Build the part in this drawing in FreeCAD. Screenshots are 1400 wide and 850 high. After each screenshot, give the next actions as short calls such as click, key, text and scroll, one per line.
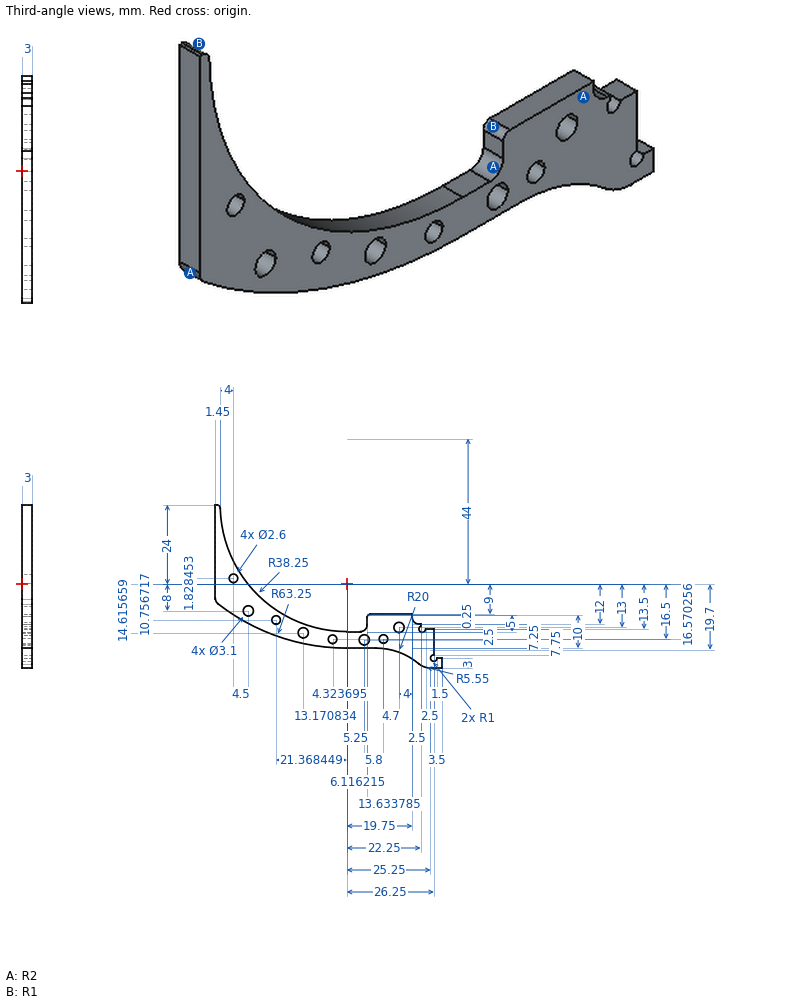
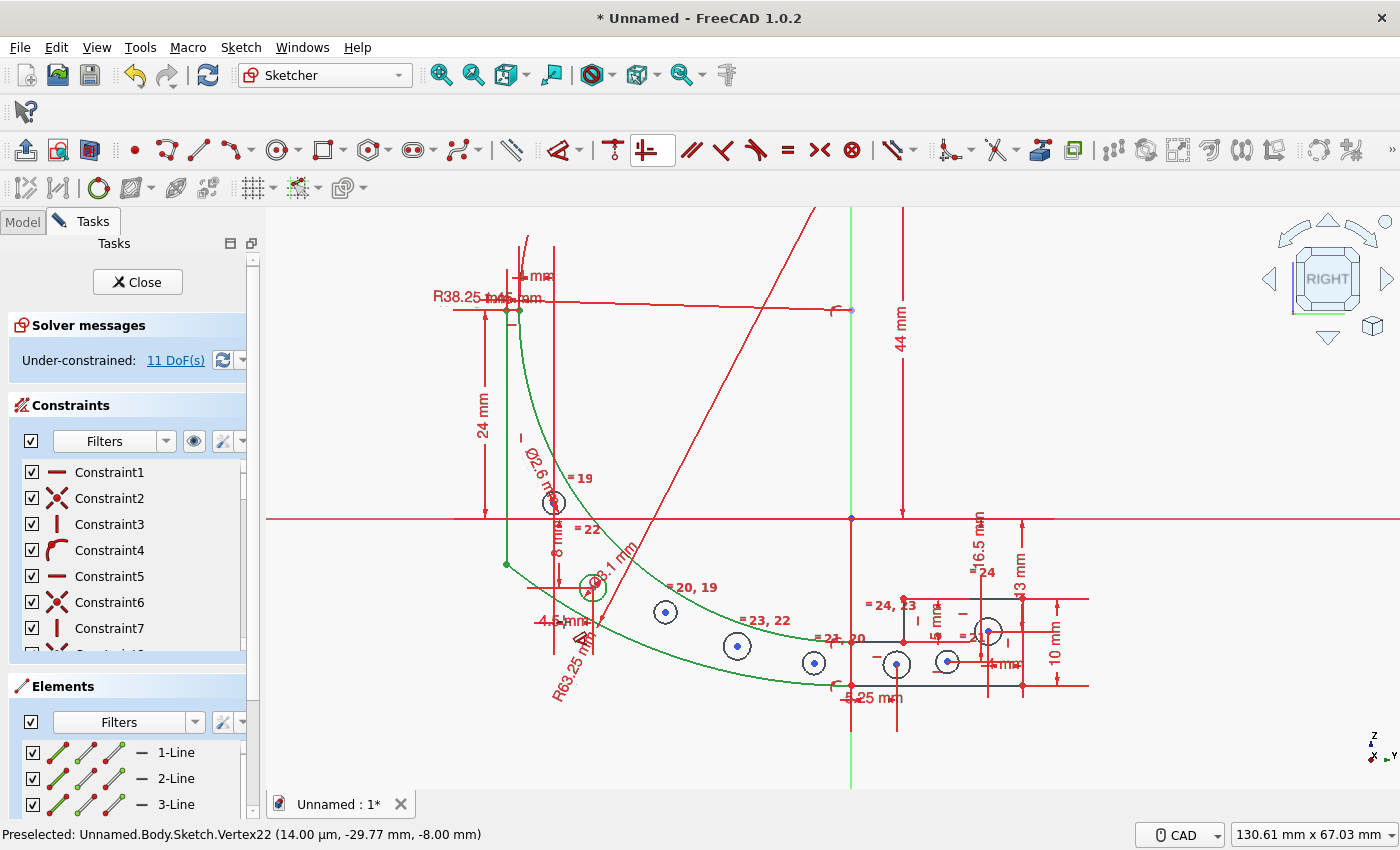
scroll(904, 642, up, 4)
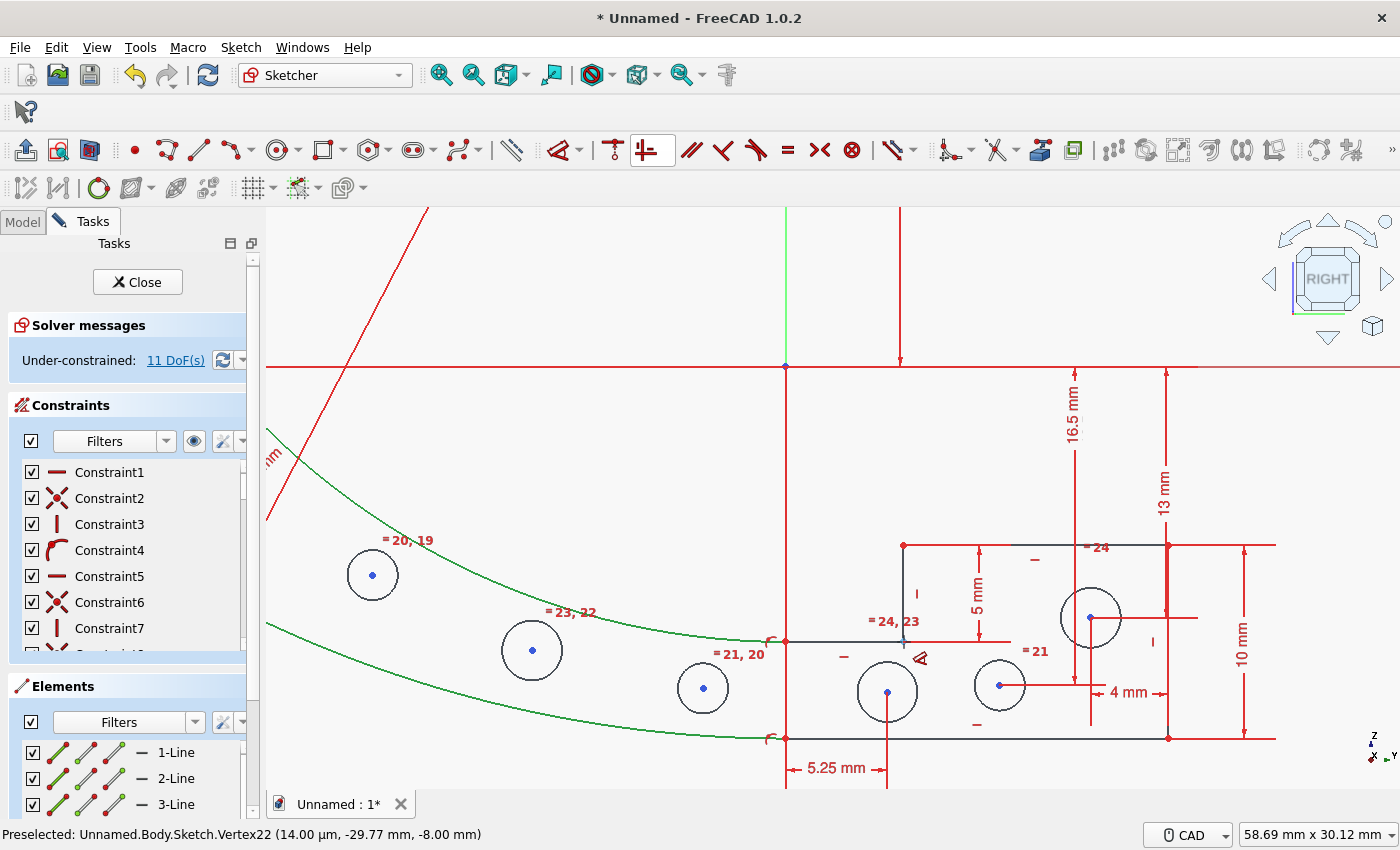
click(903, 642)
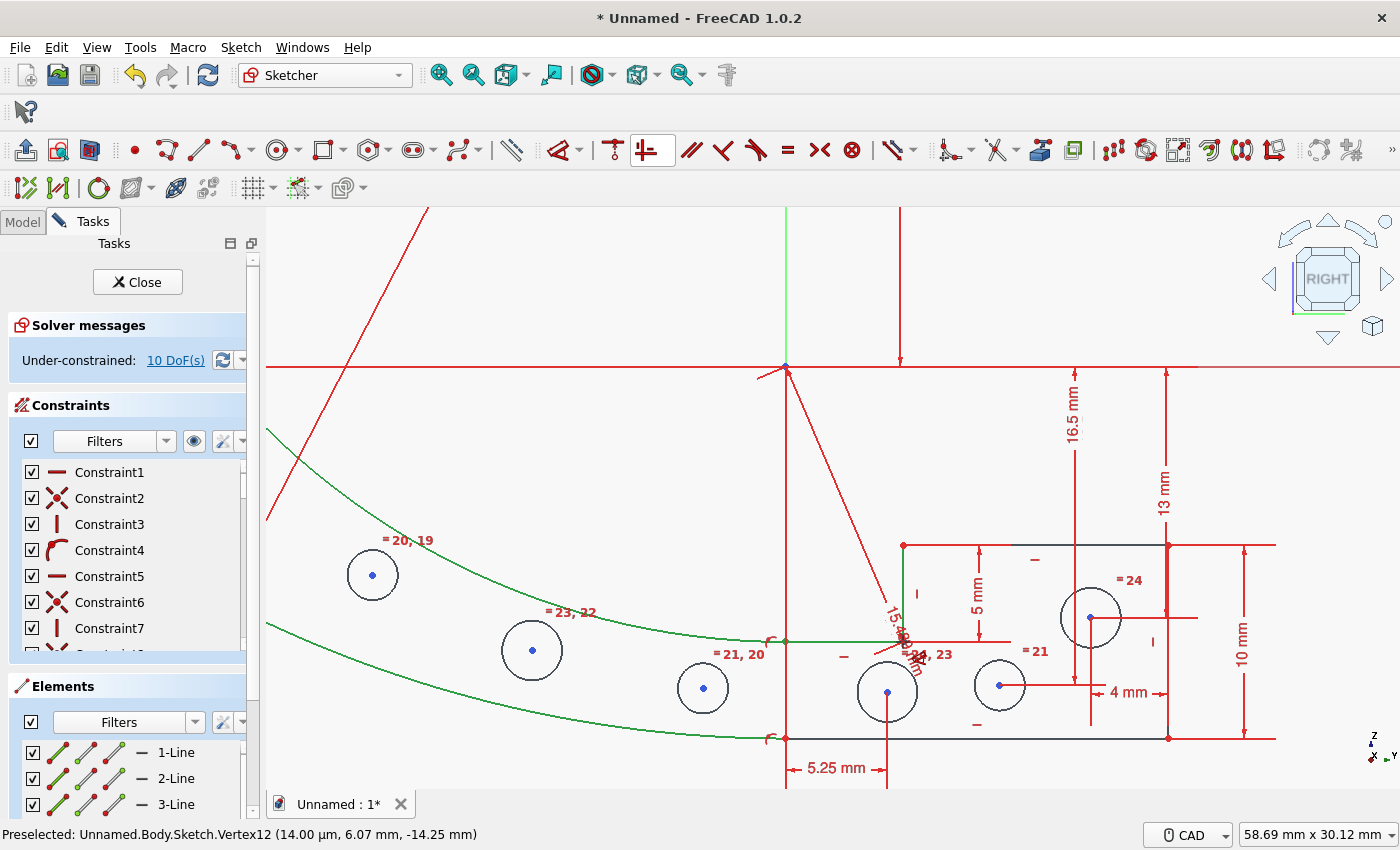
click(887, 692)
click(937, 667)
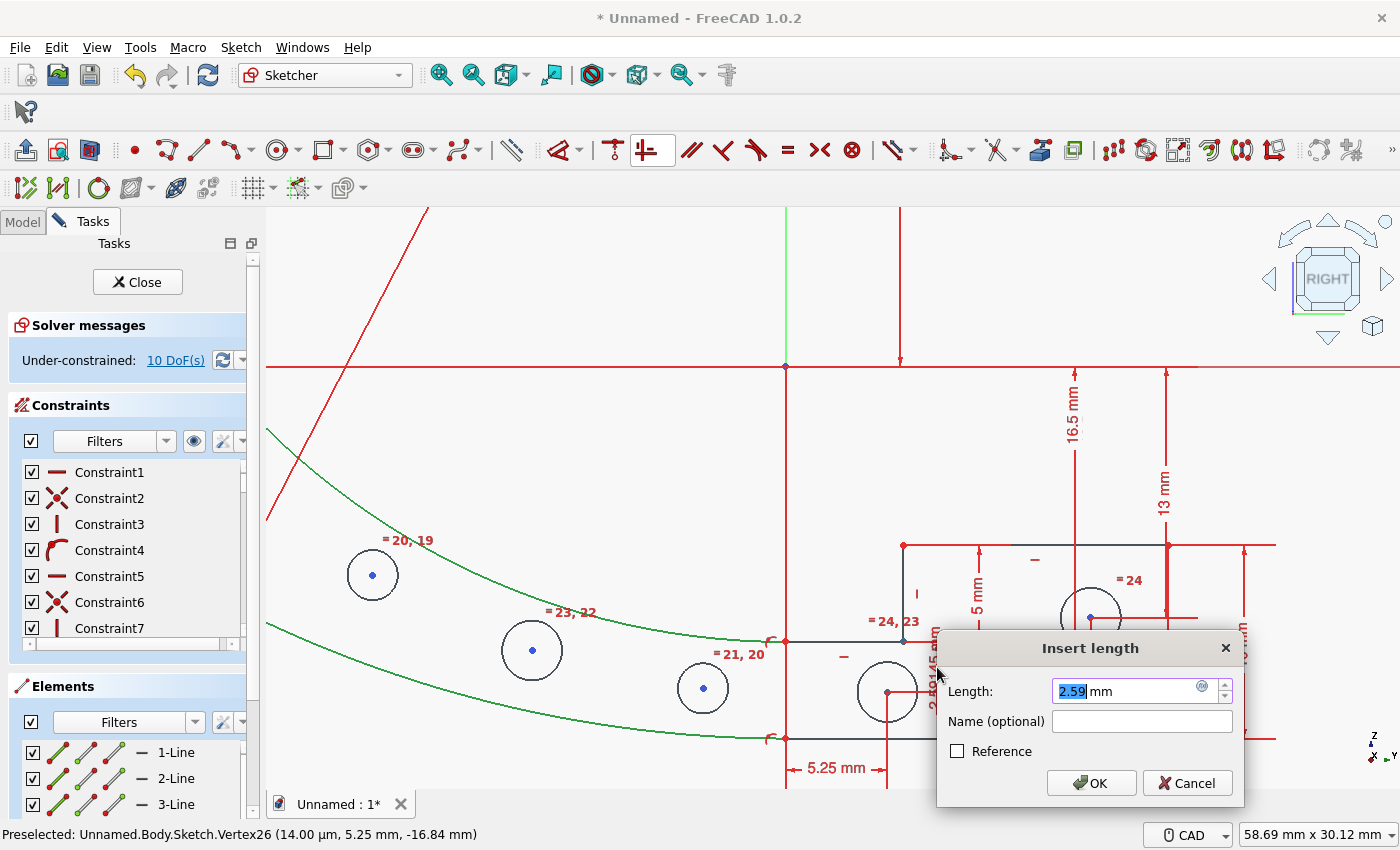
text(2.5)
key(Return)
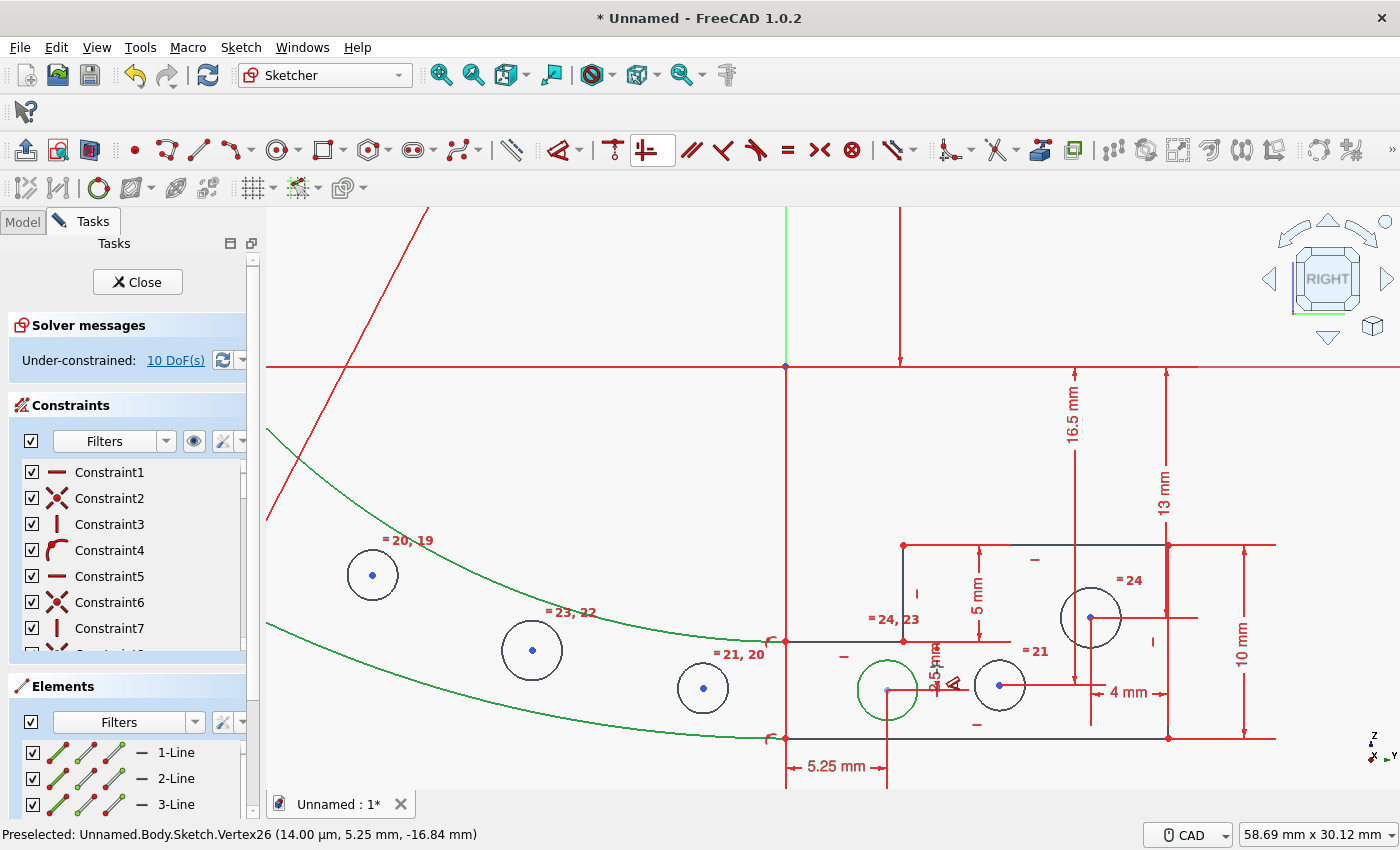
click(887, 690)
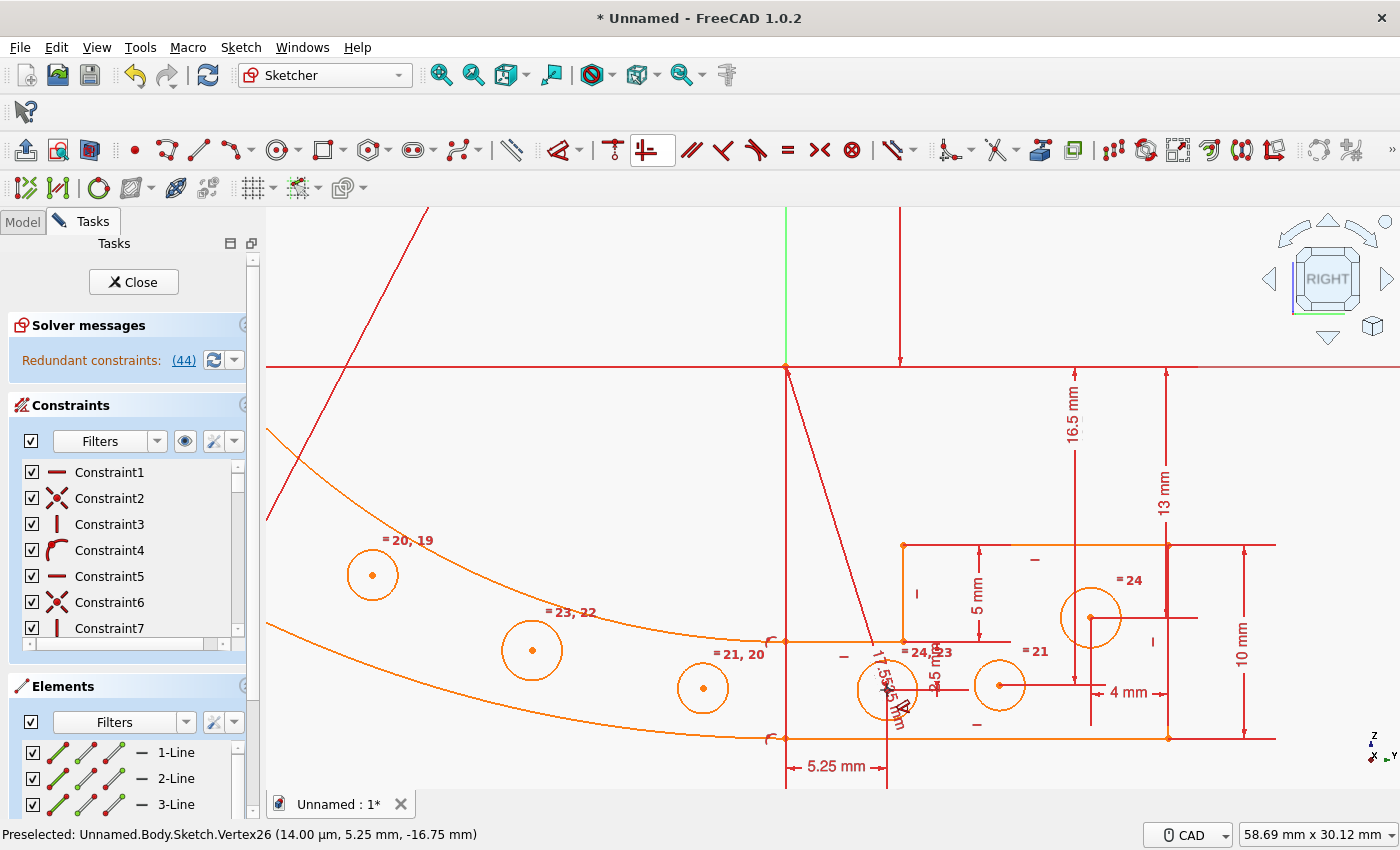
click(1000, 685)
click(944, 724)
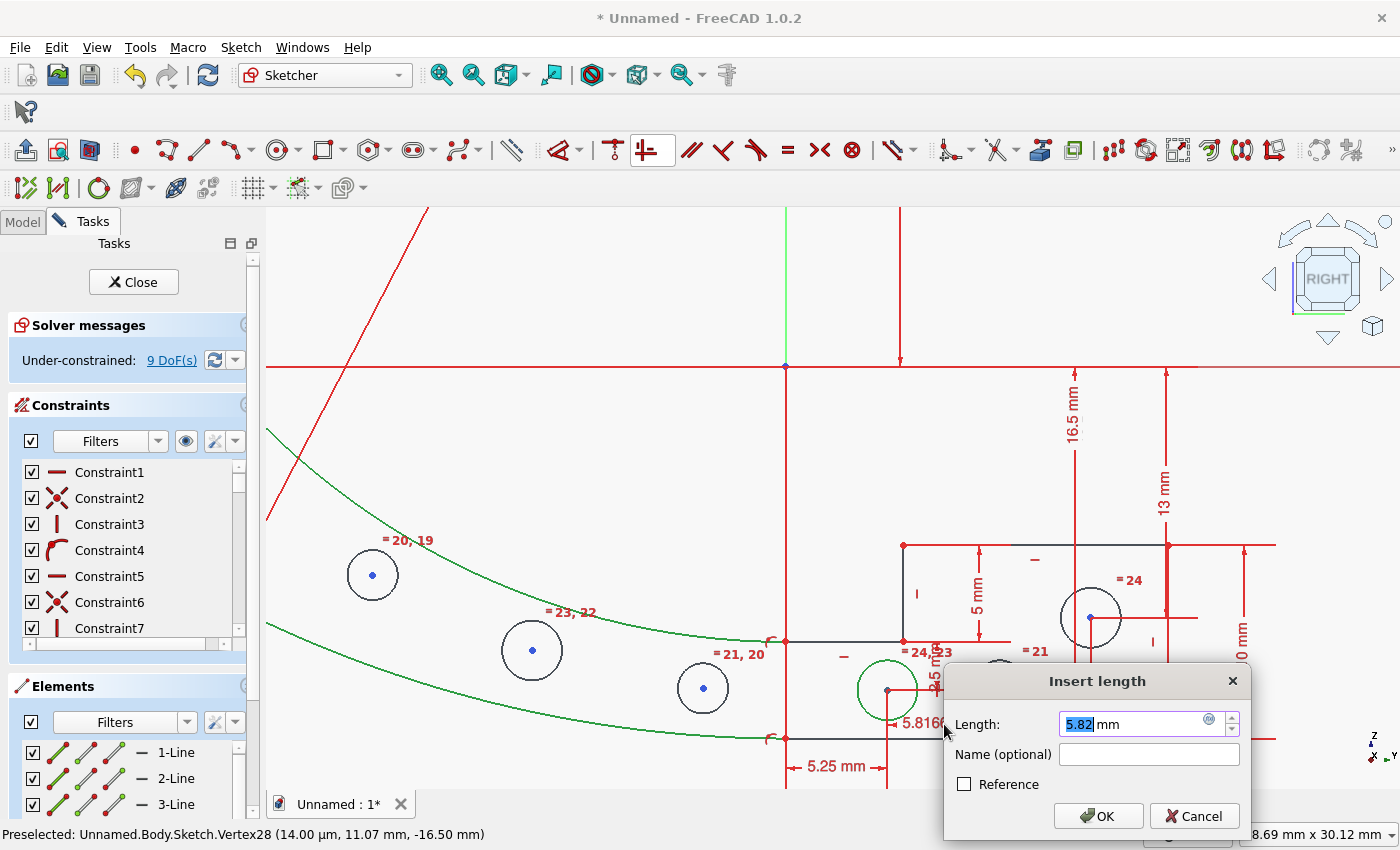
text(5.8)
key(Return)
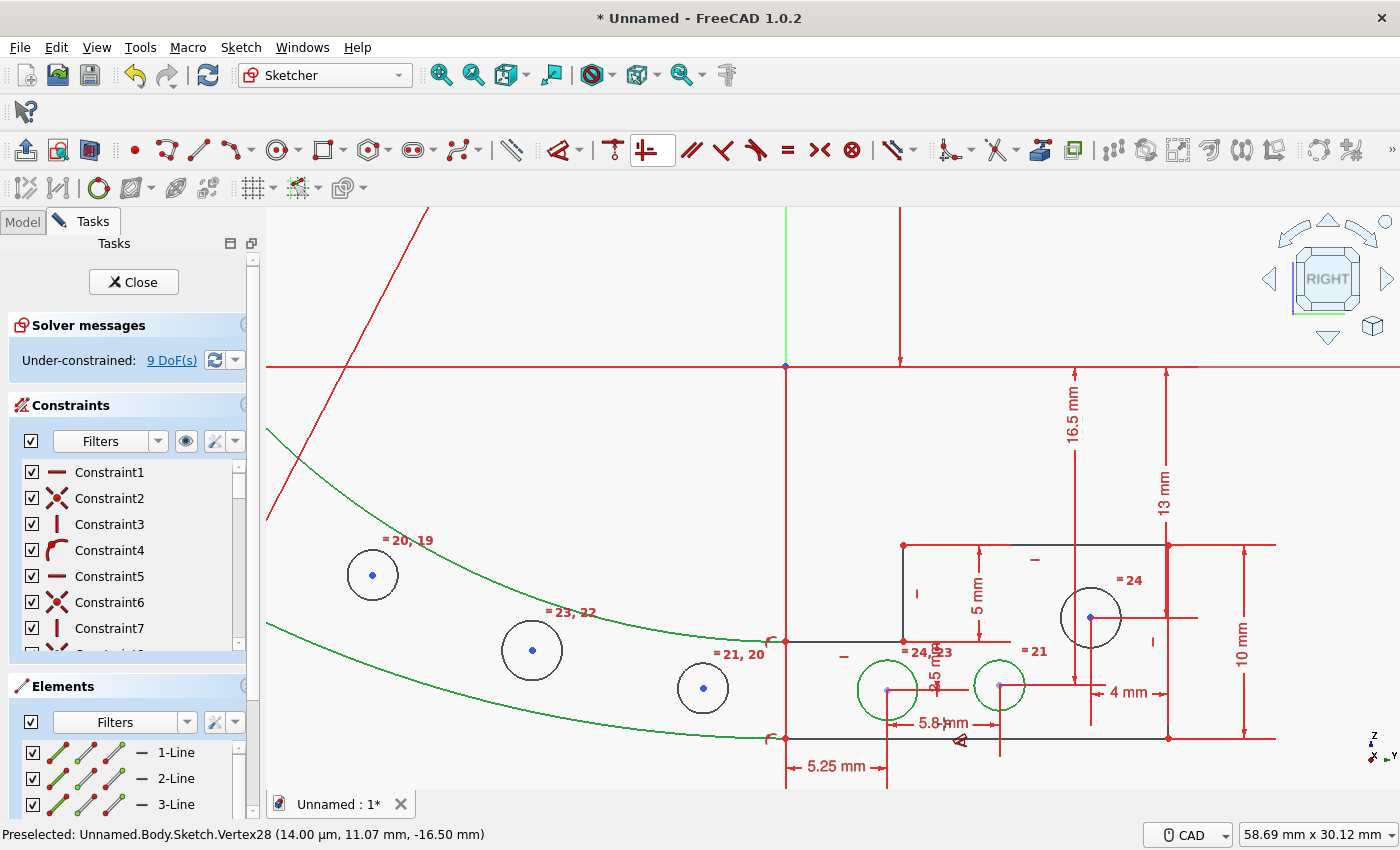
click(1091, 618)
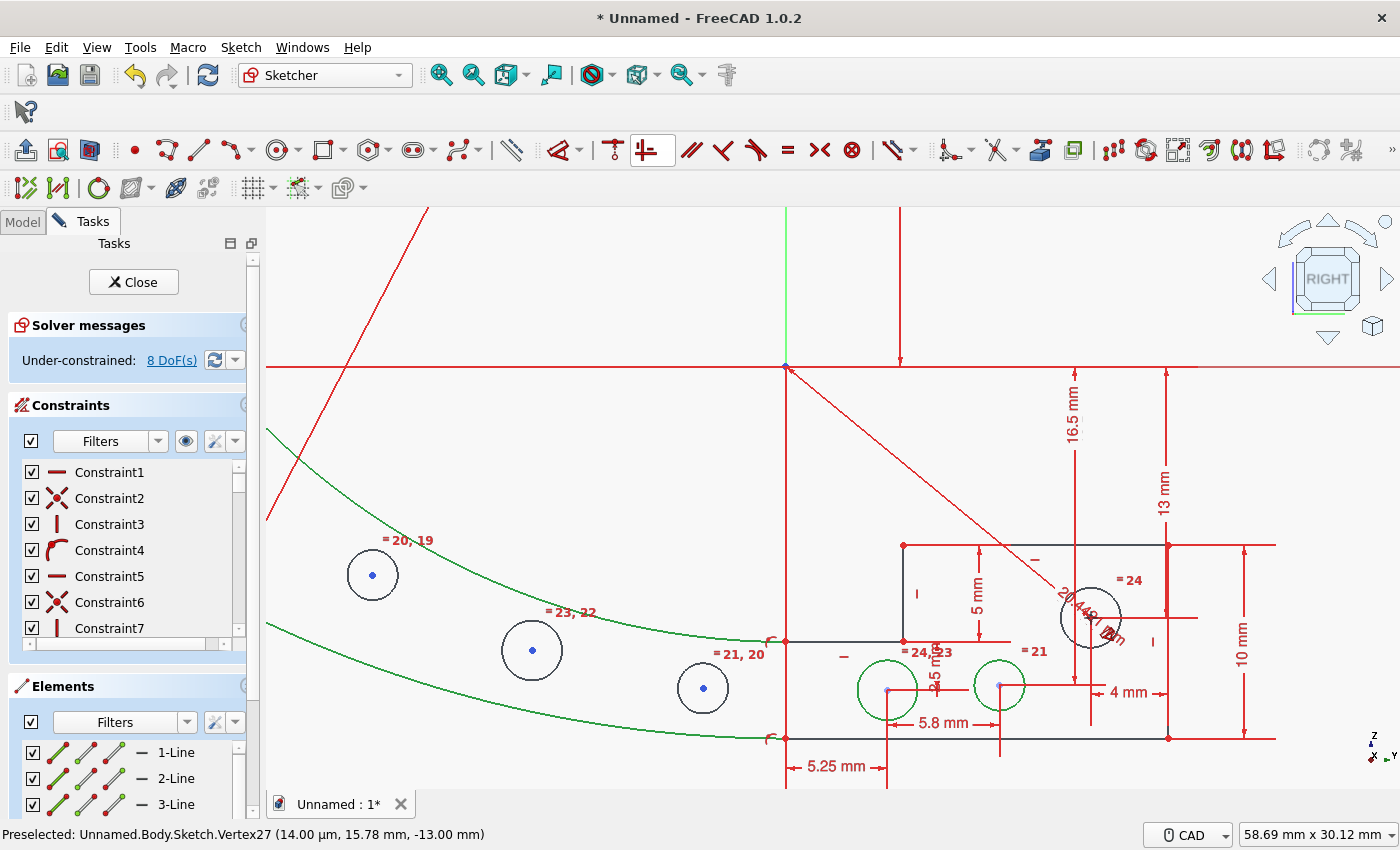
click(1000, 685)
click(1045, 719)